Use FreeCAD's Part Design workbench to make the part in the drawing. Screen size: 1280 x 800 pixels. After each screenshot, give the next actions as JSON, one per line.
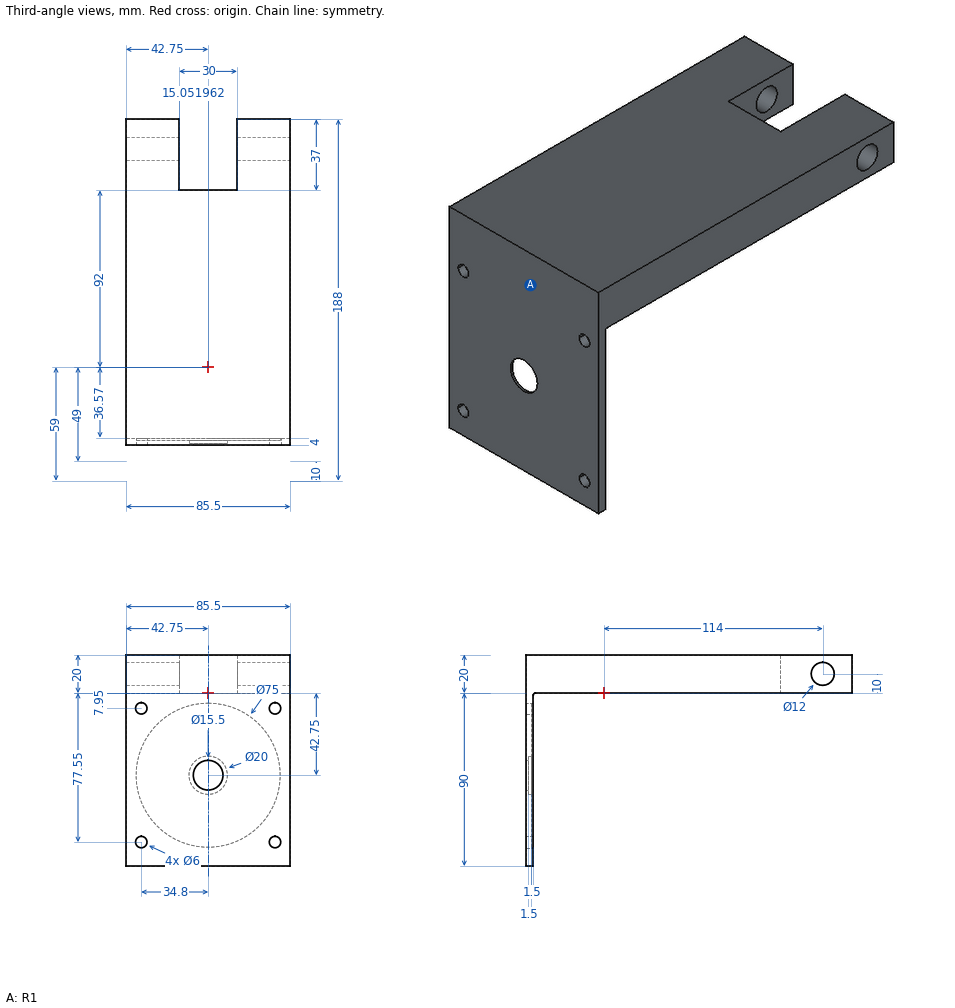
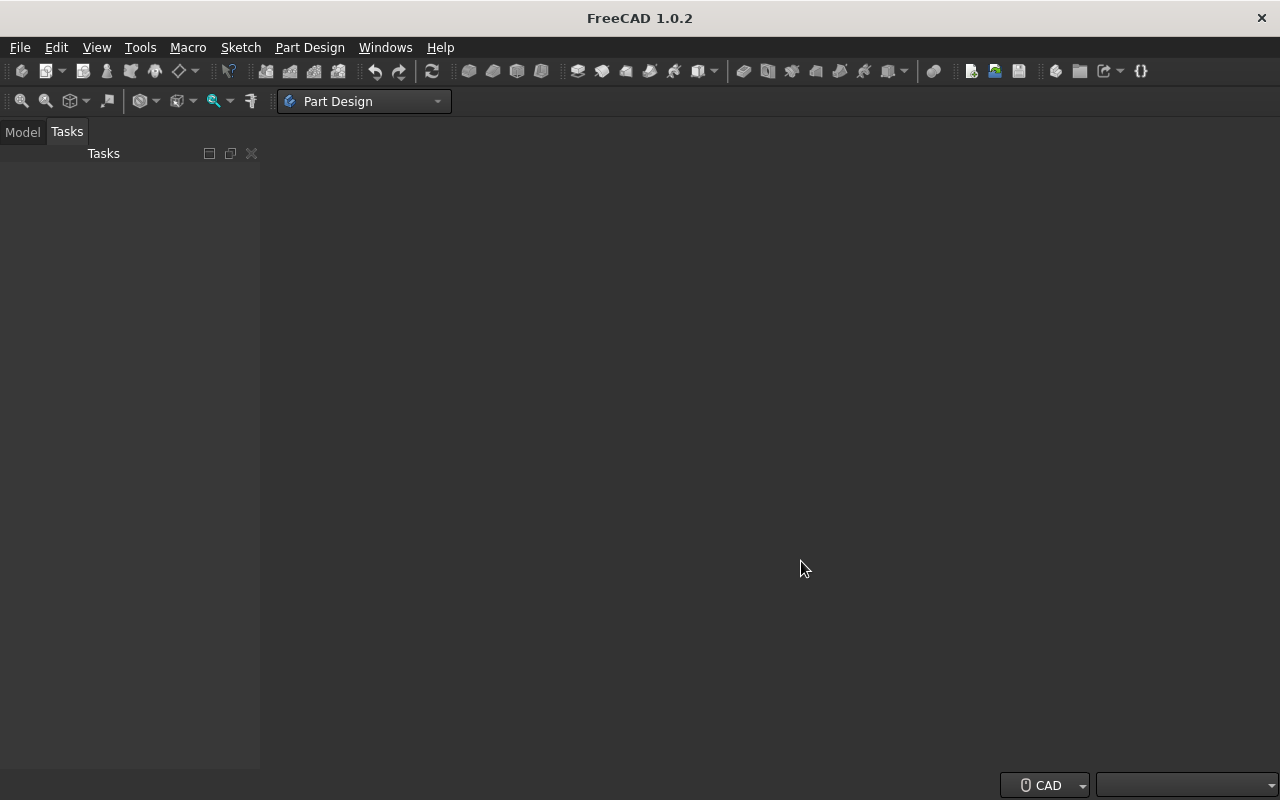
{"action": "key", "text": "ctrl+n"}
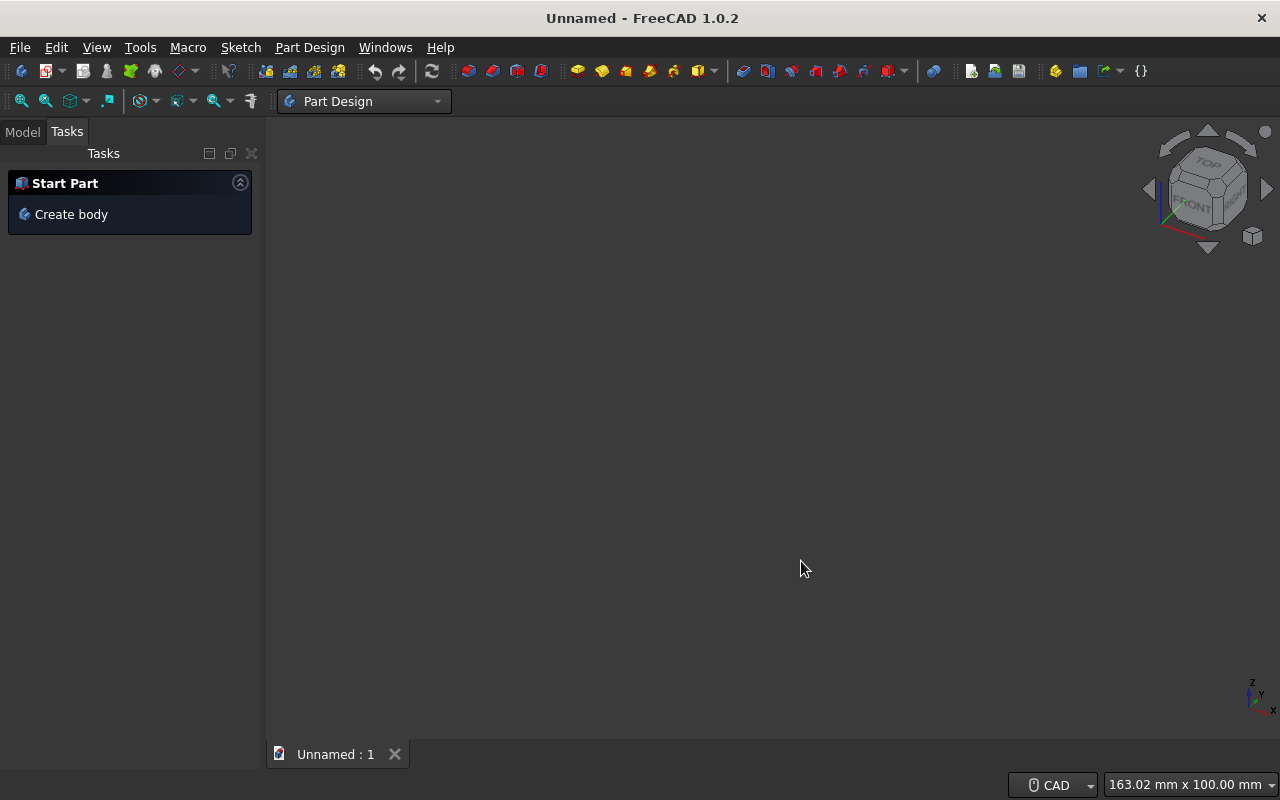
{"action": "left_click", "coordinate": [46, 72]}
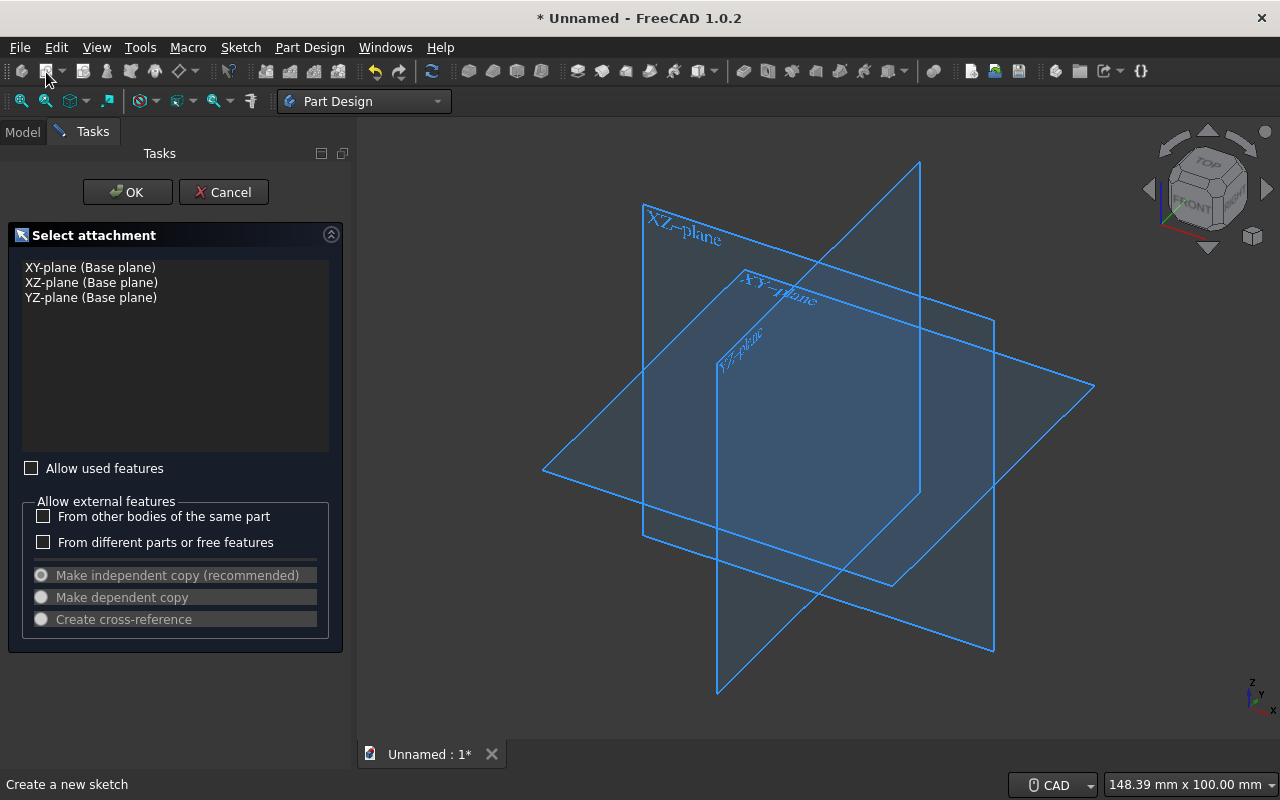
{"action": "left_click", "coordinate": [82, 268]}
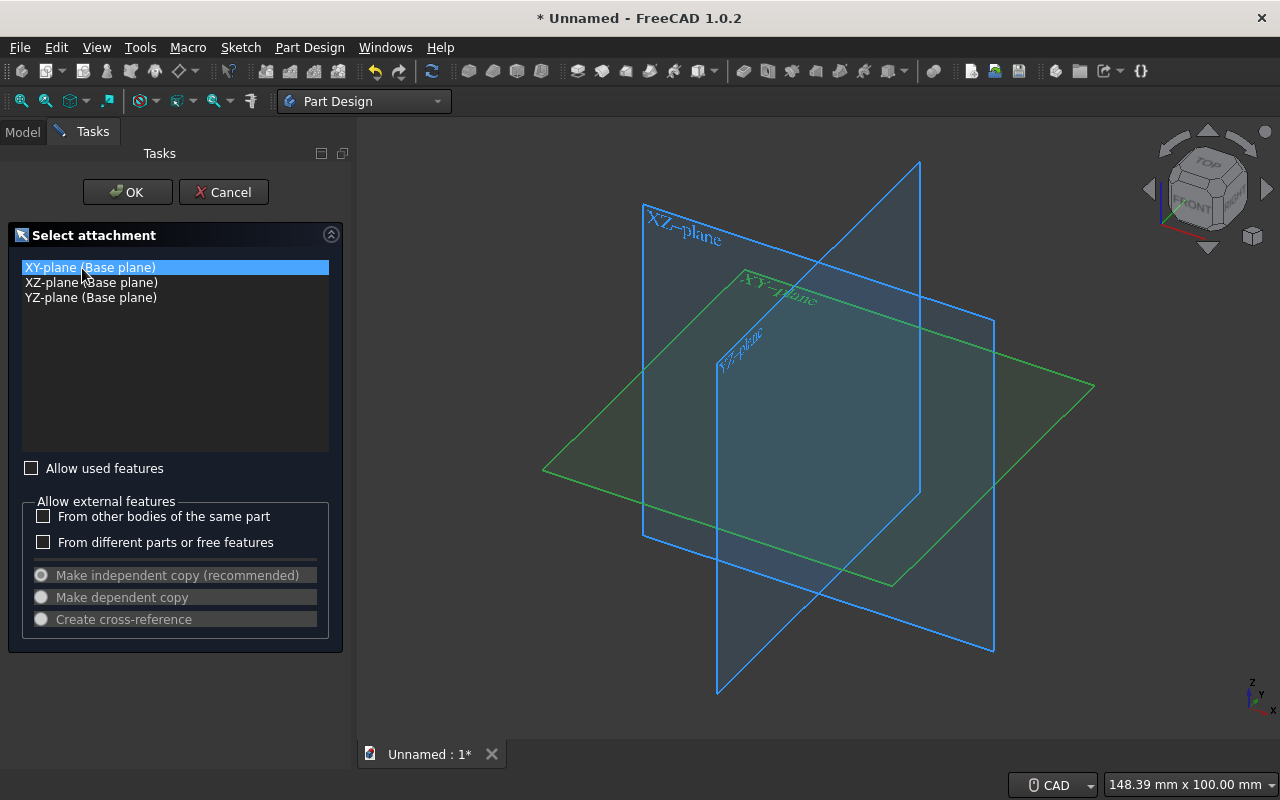
{"action": "left_click", "coordinate": [128, 192]}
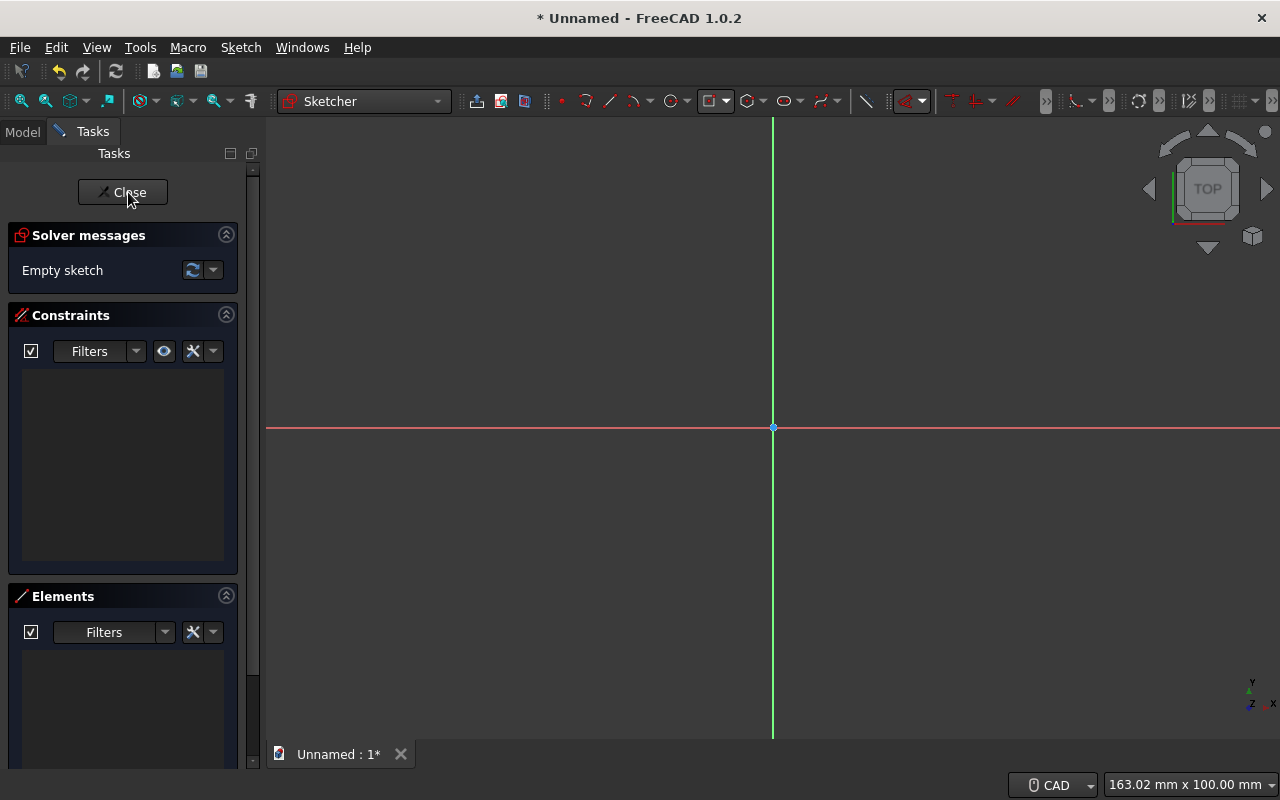
{"action": "scroll", "coordinate": [665, 555], "scroll_direction": "down", "scroll_amount": 5}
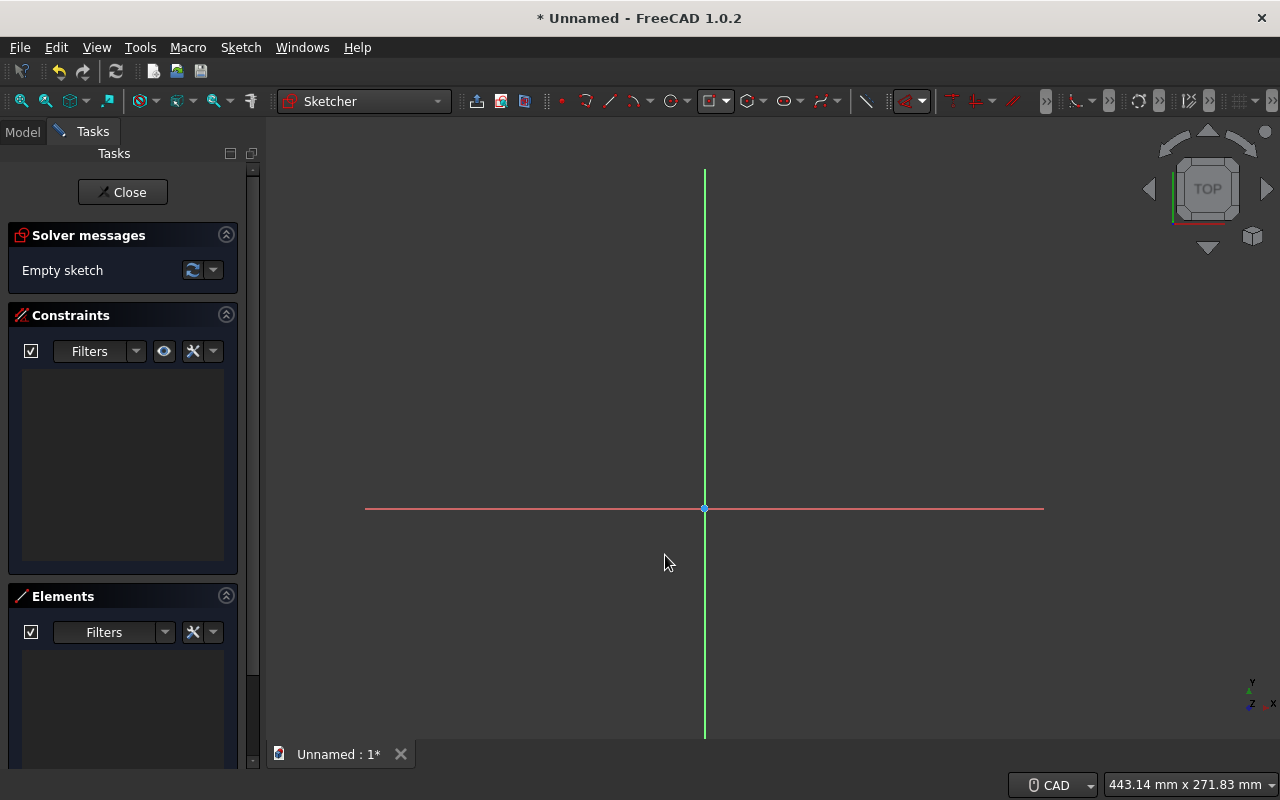
{"action": "key", "text": "g r"}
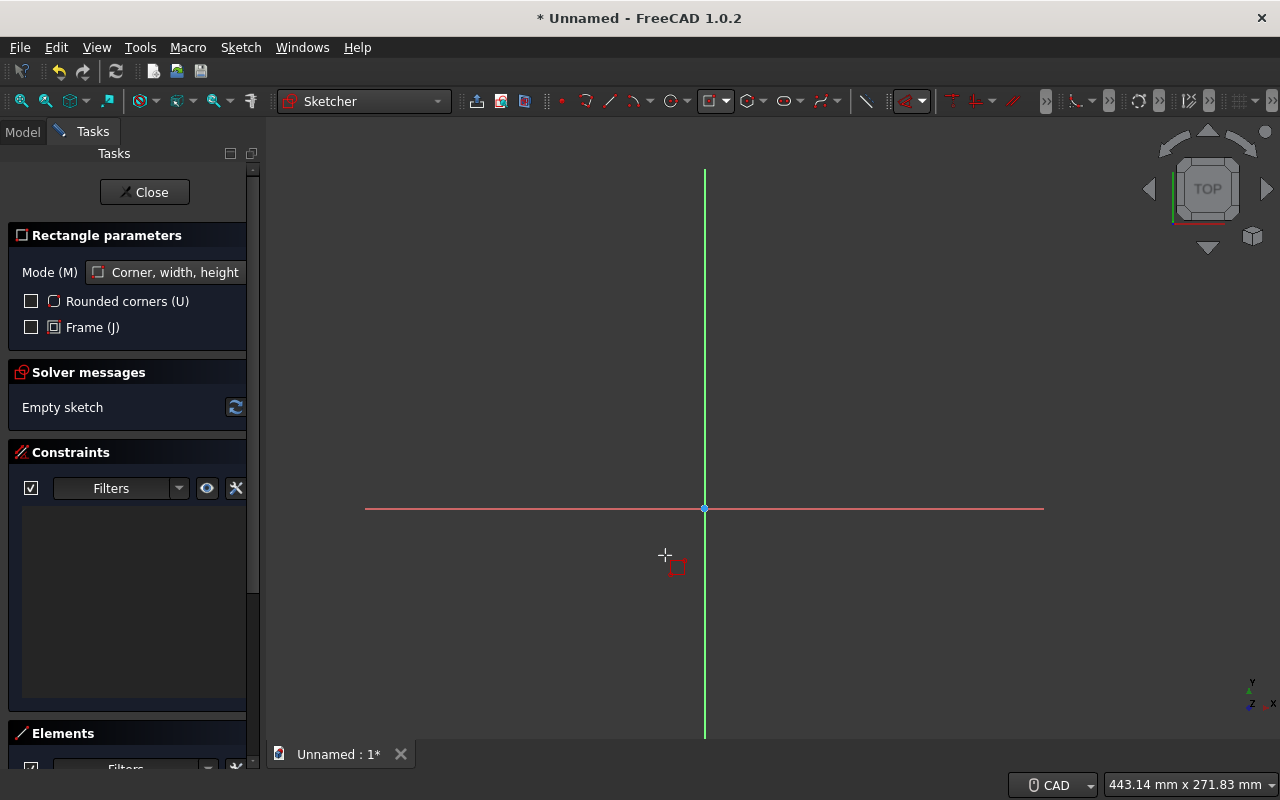
{"action": "left_click", "coordinate": [607, 214]}
{"action": "mouse_move", "coordinate": [803, 644]}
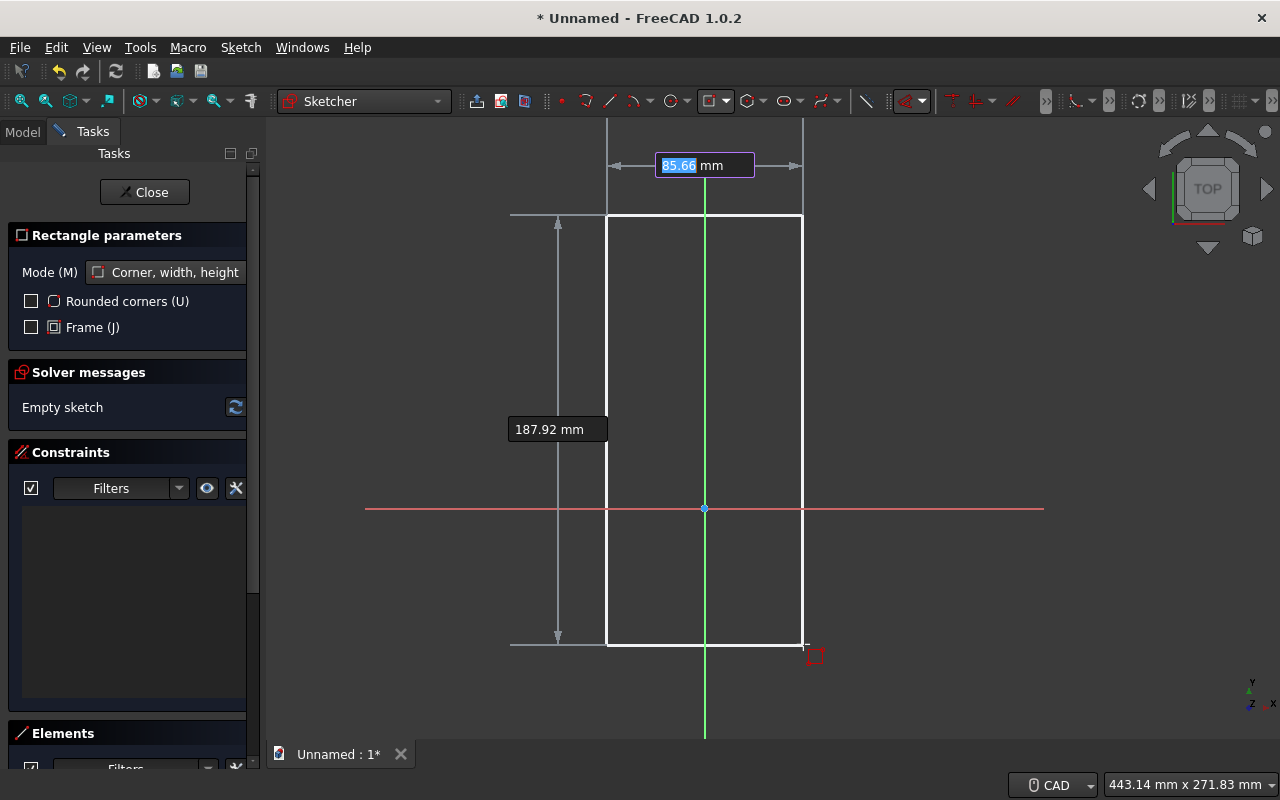
{"action": "type", "text": "85.5"}
{"action": "key", "text": "Tab"}
{"action": "type", "text": "188"}
{"action": "key", "text": "Return"}
{"action": "key", "text": "Escape"}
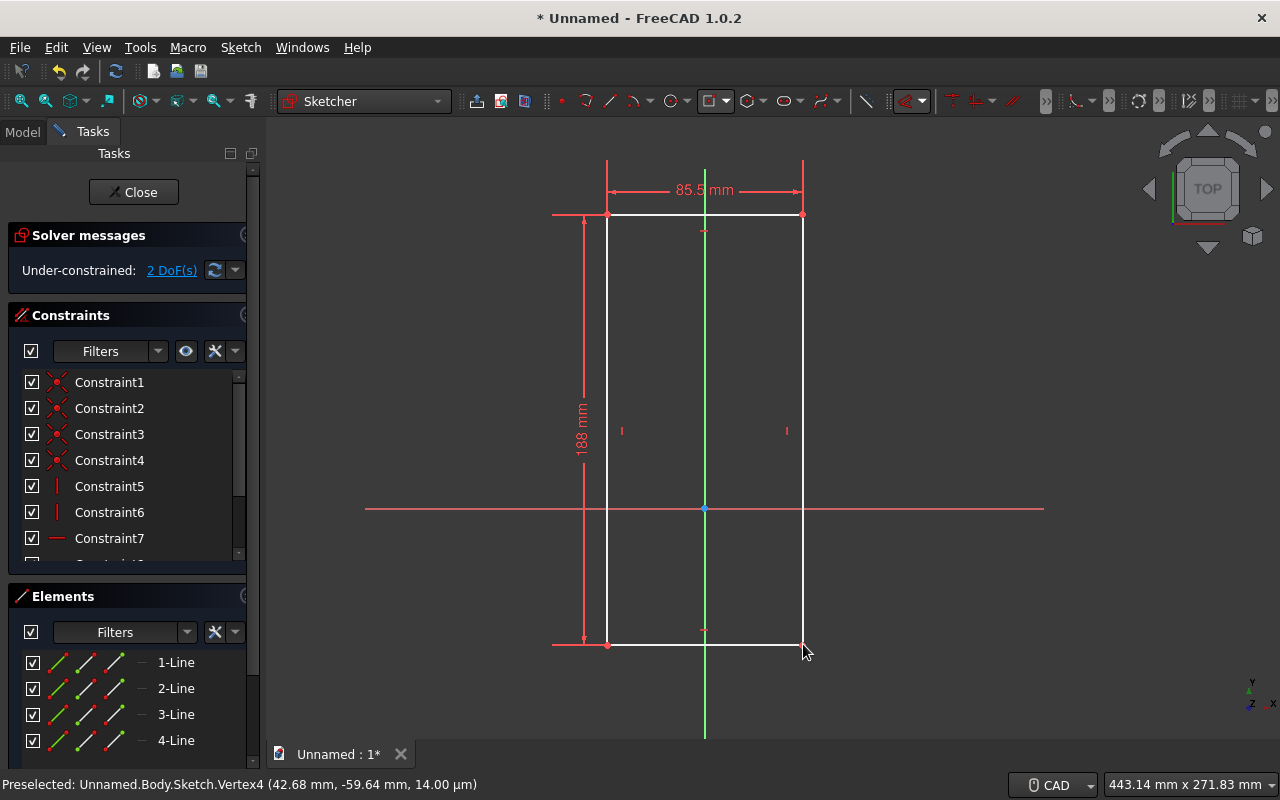
{"action": "key", "text": "d"}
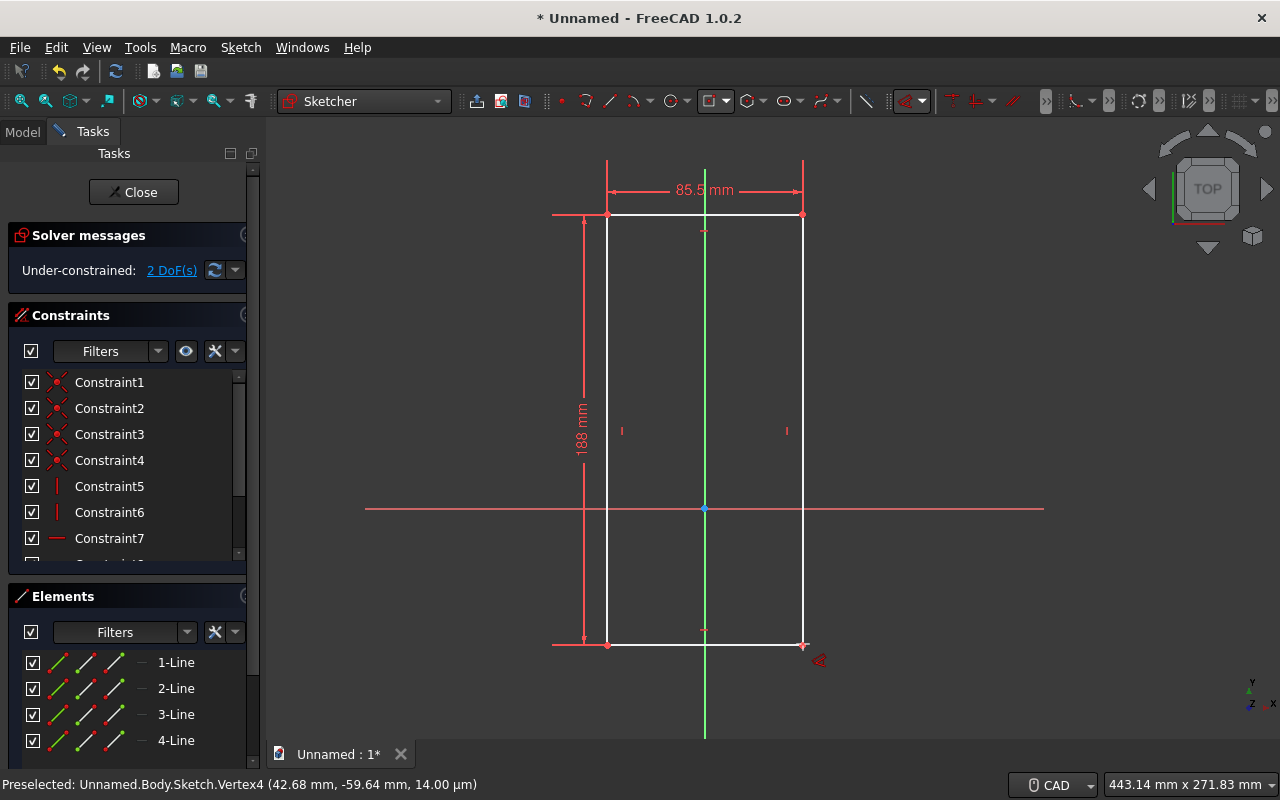
{"action": "left_click", "coordinate": [607, 645]}
{"action": "left_click", "coordinate": [573, 577]}